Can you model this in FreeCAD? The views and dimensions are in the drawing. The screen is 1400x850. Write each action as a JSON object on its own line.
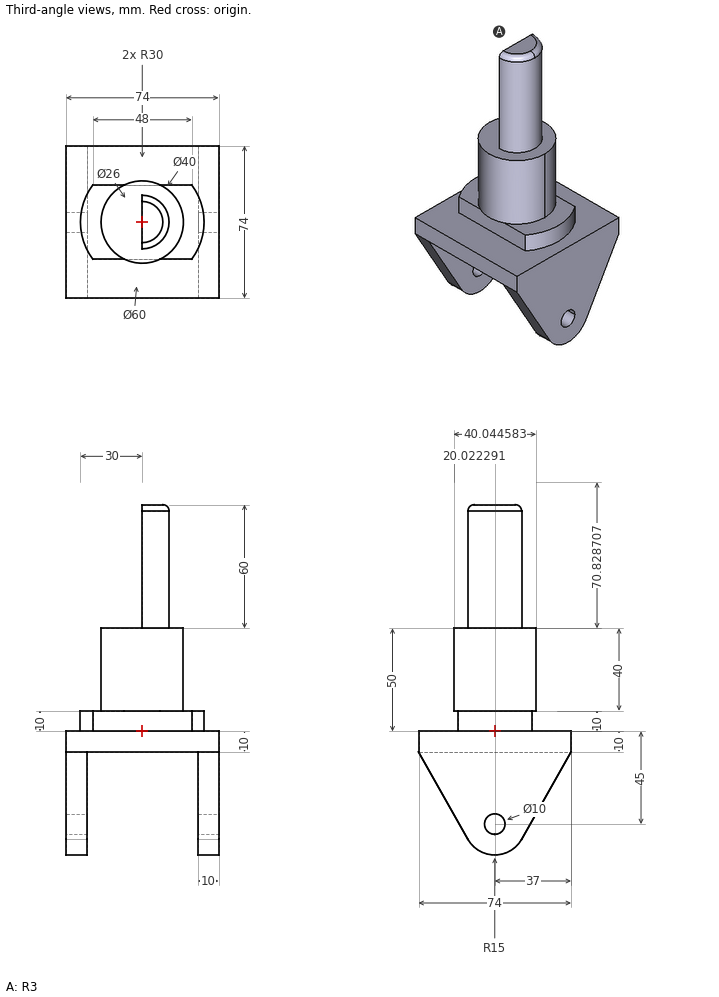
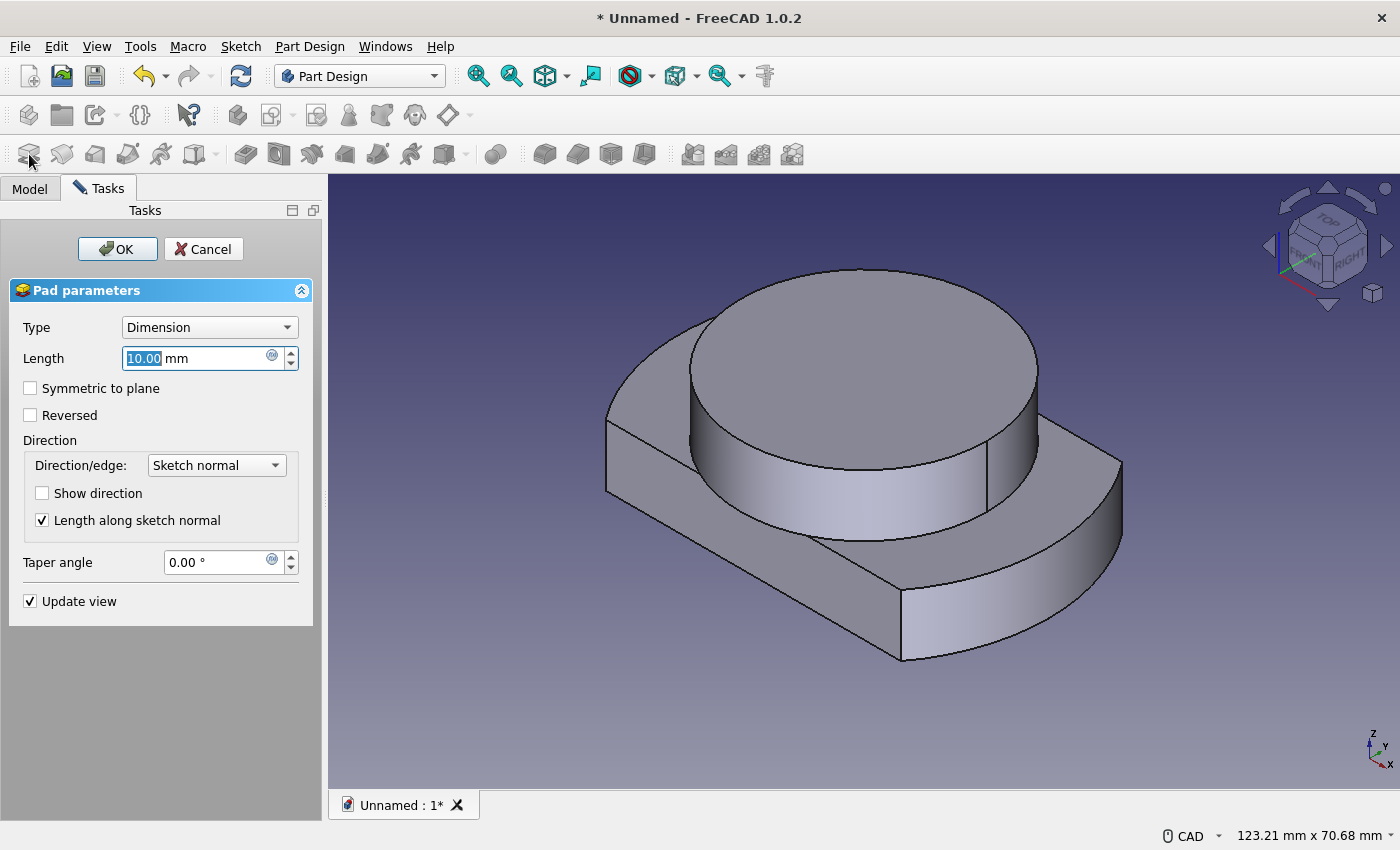
{"action": "type", "text": "40"}
{"action": "key", "text": "Tab"}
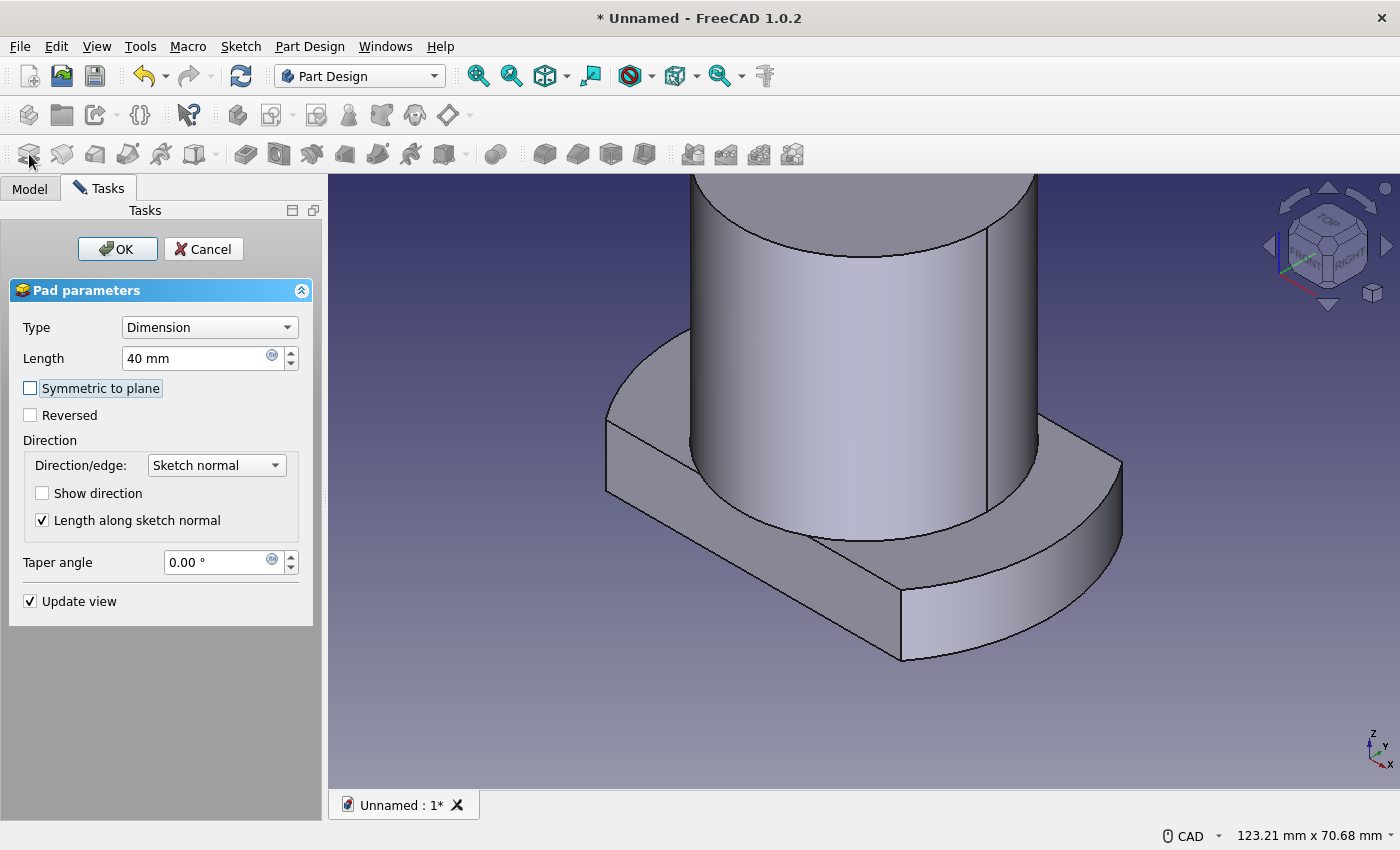
{"action": "left_click", "coordinate": [118, 249]}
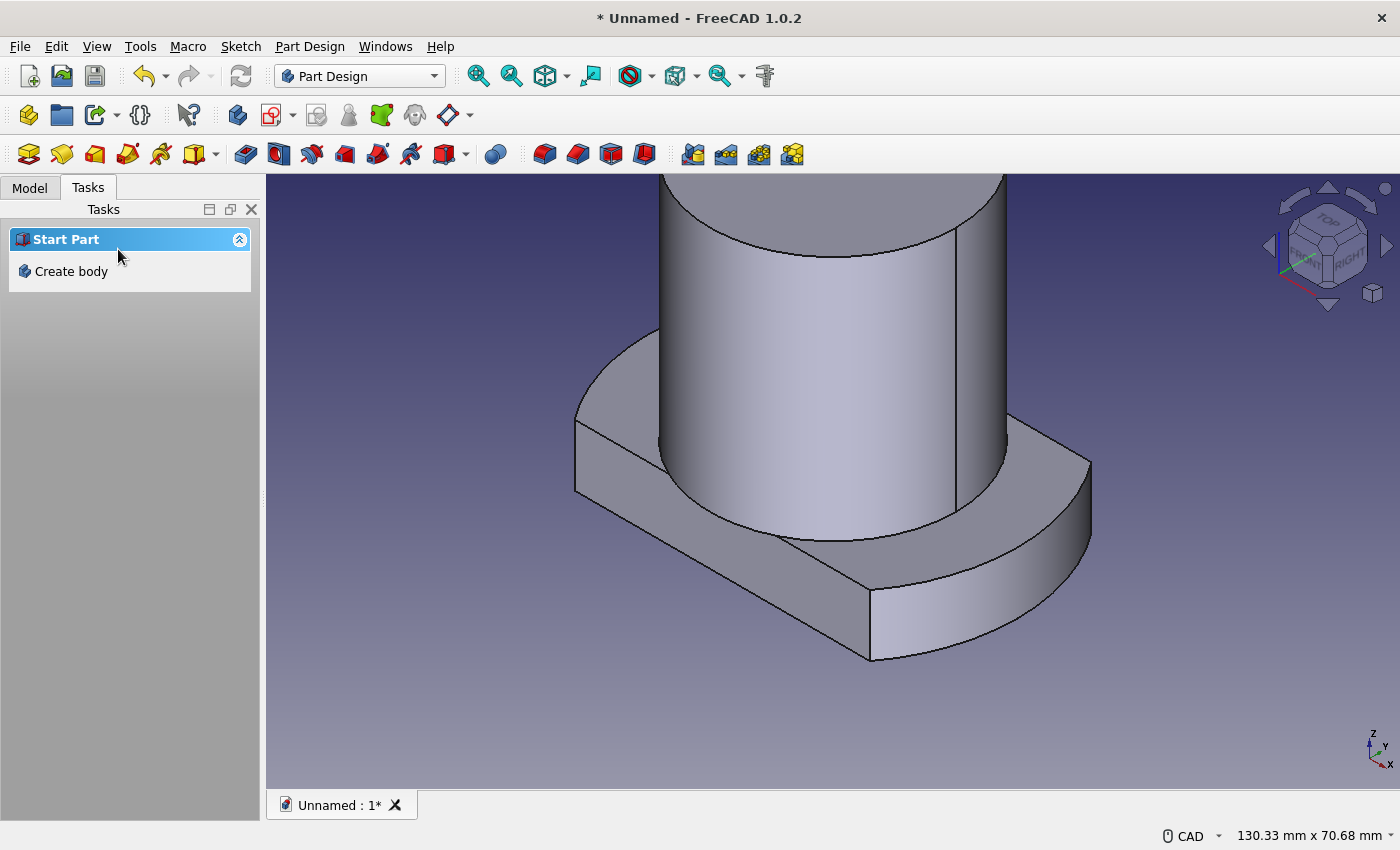
{"action": "left_click", "coordinate": [479, 76]}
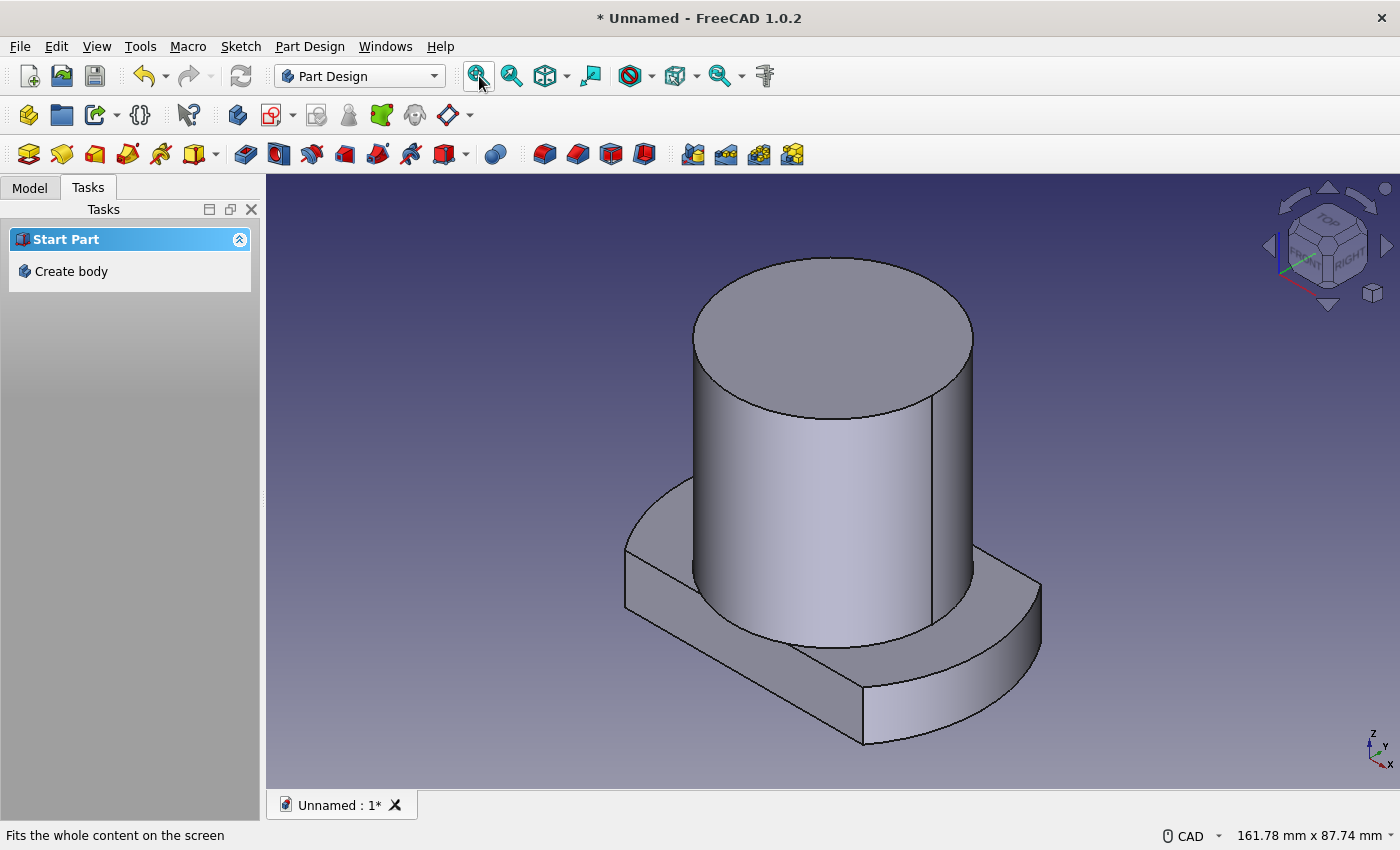
{"action": "left_click", "coordinate": [833, 337]}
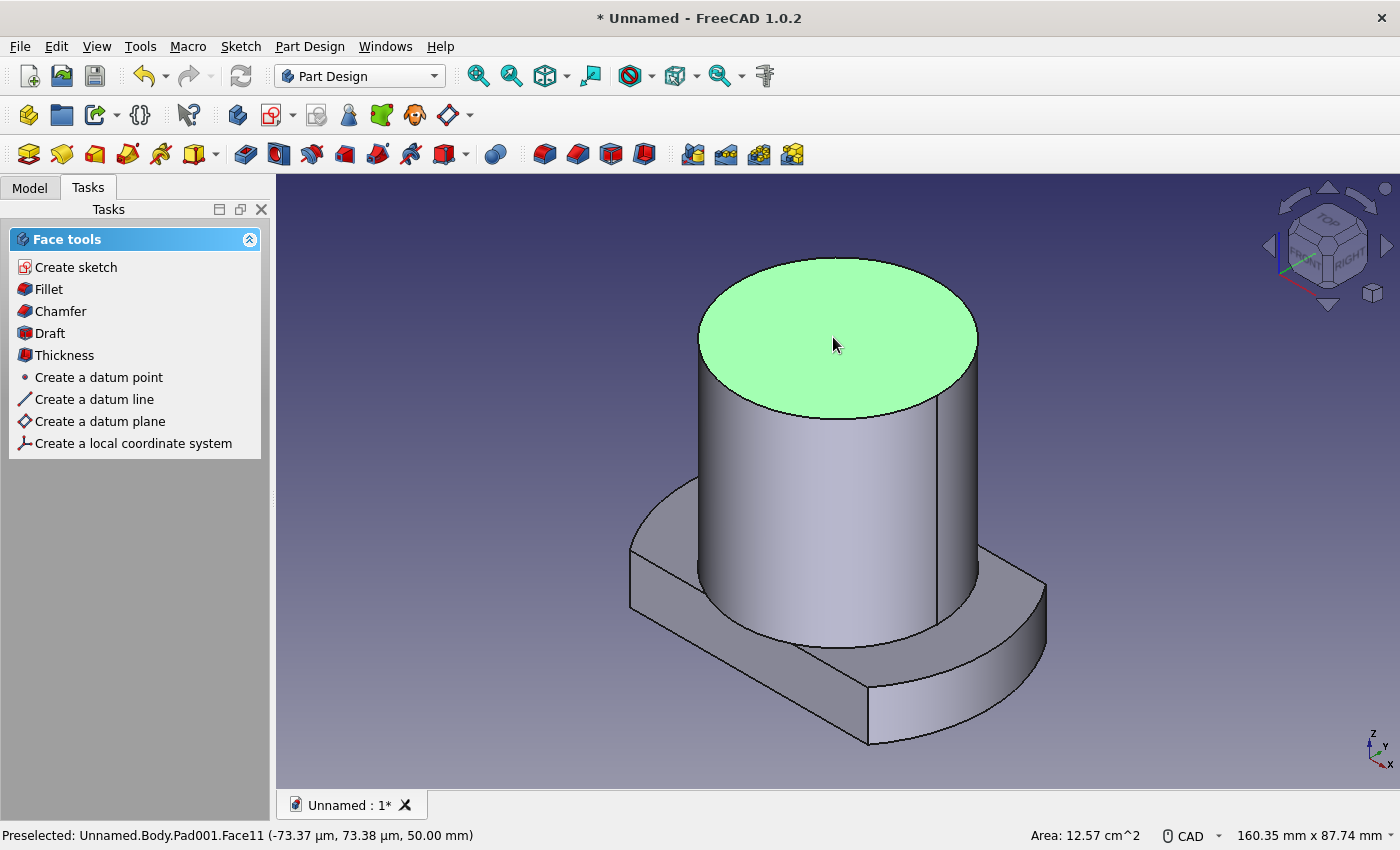
{"action": "left_click", "coordinate": [270, 116]}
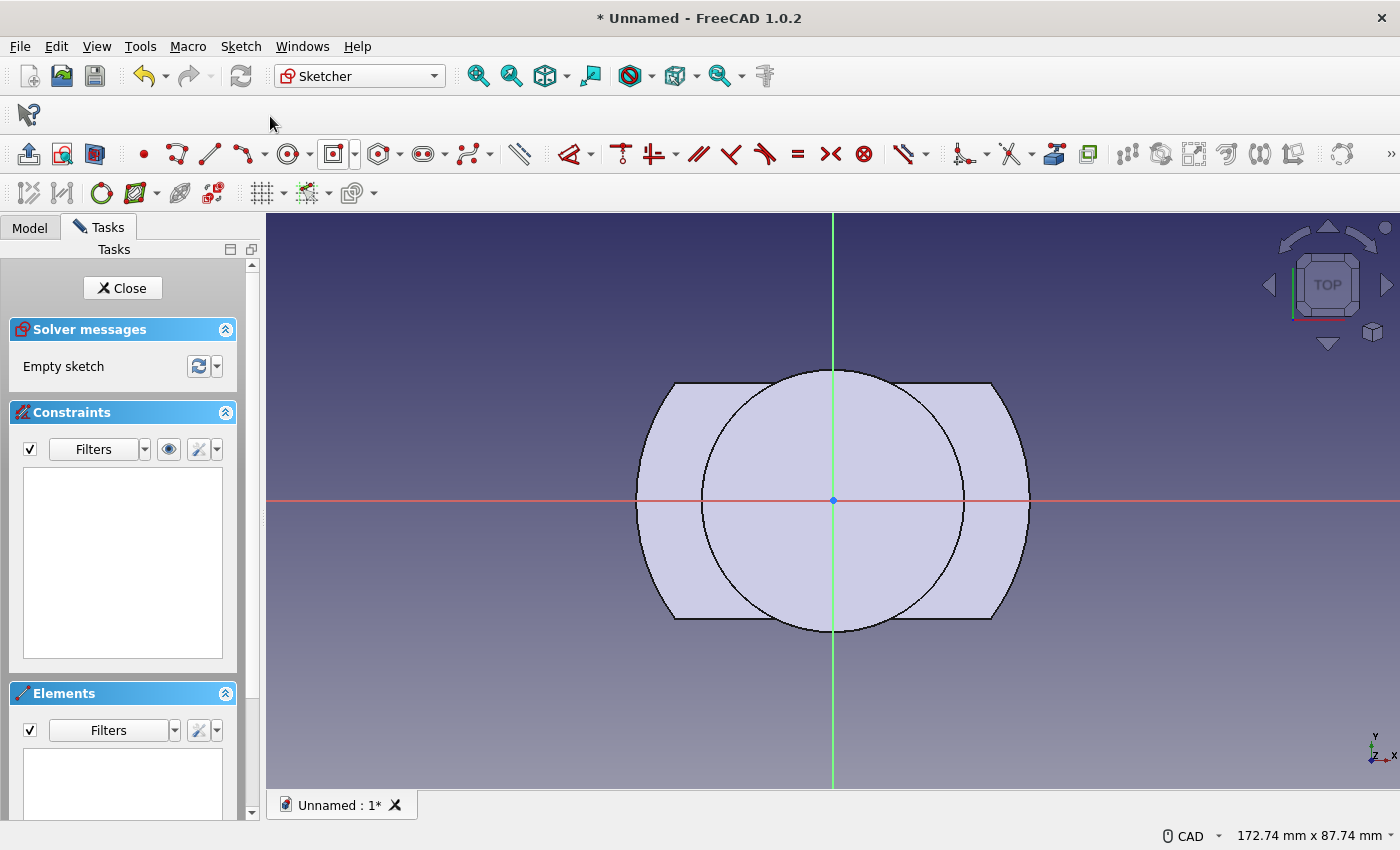
{"action": "scroll", "coordinate": [889, 501], "scroll_direction": "up", "scroll_amount": 4}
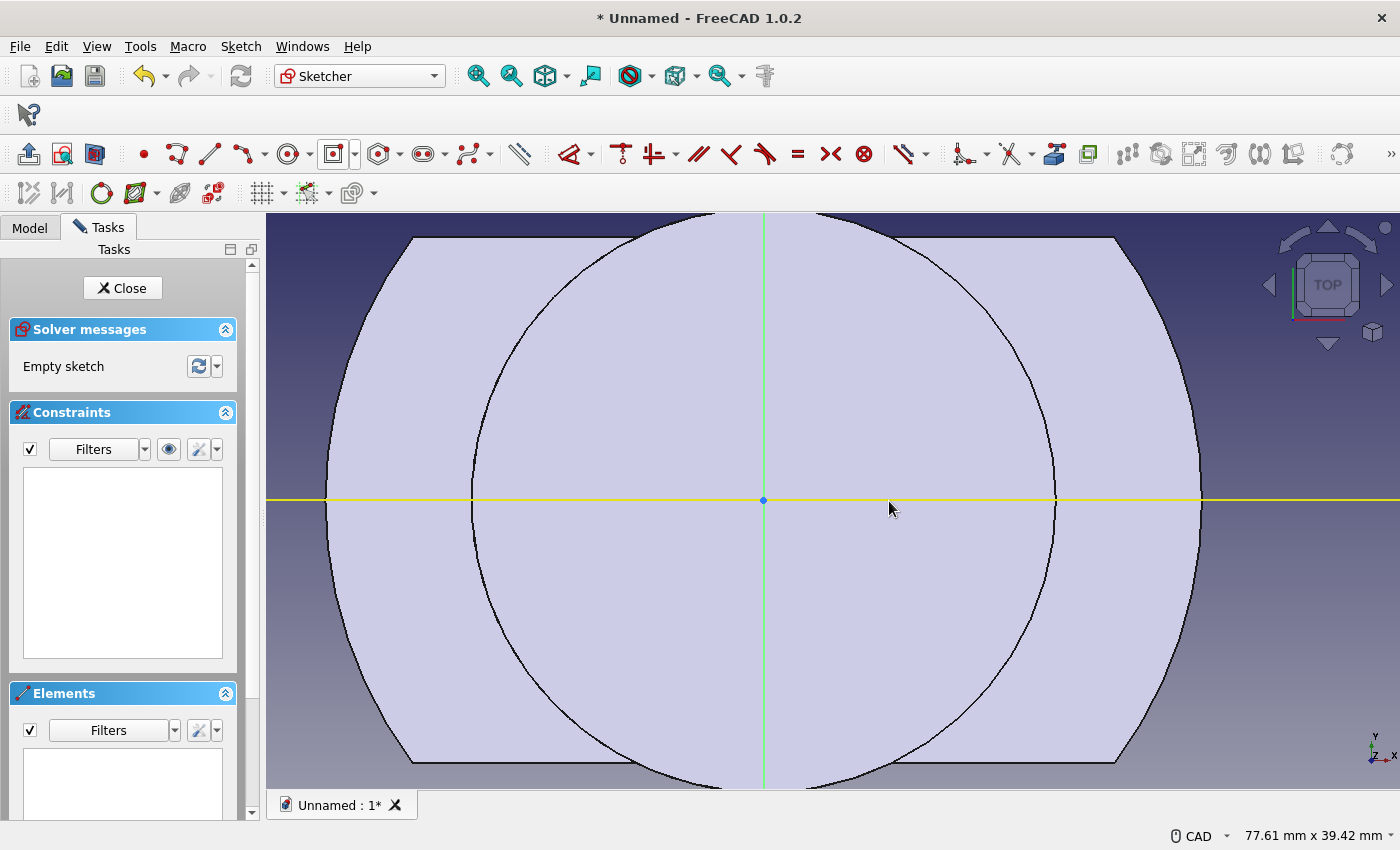
{"action": "key", "text": "g c"}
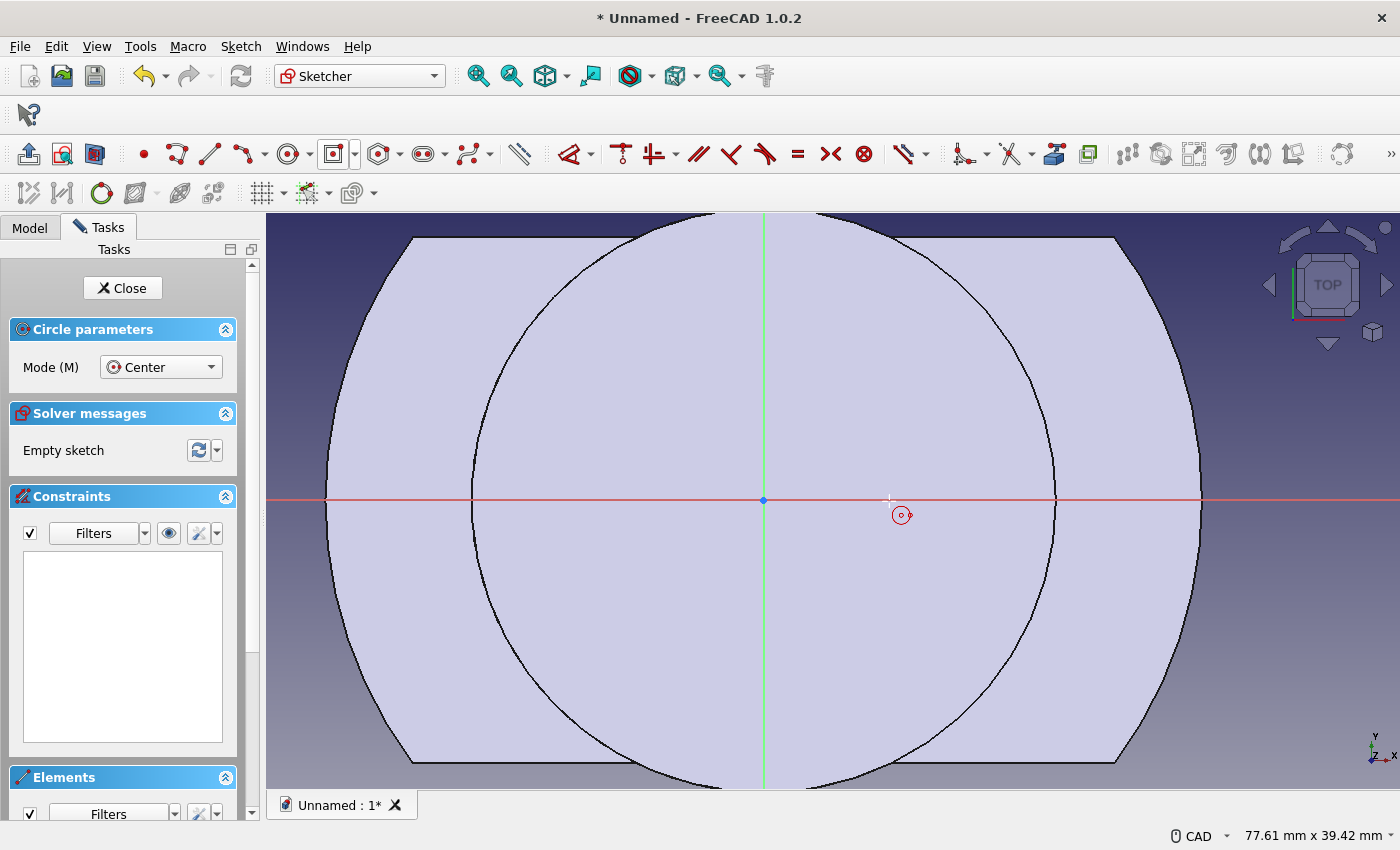
{"action": "left_click", "coordinate": [764, 500]}
{"action": "mouse_move", "coordinate": [898, 366]}